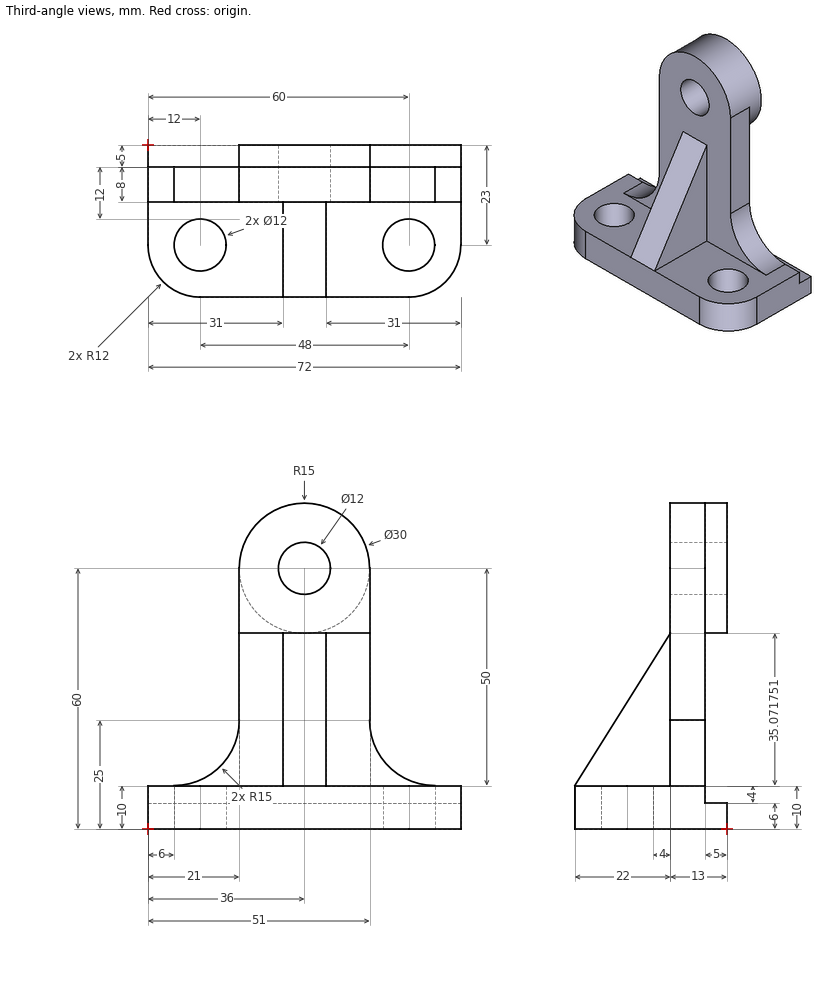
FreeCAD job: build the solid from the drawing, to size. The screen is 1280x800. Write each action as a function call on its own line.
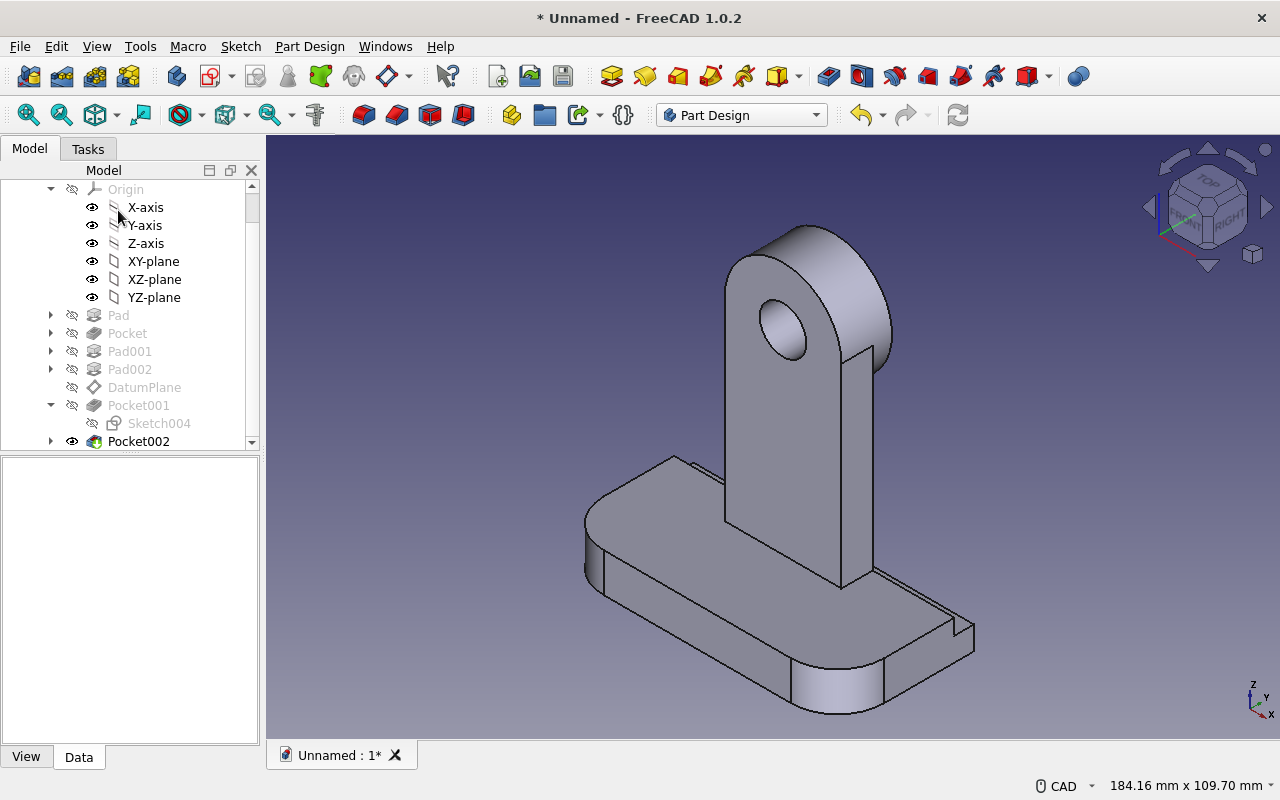
click(783, 449)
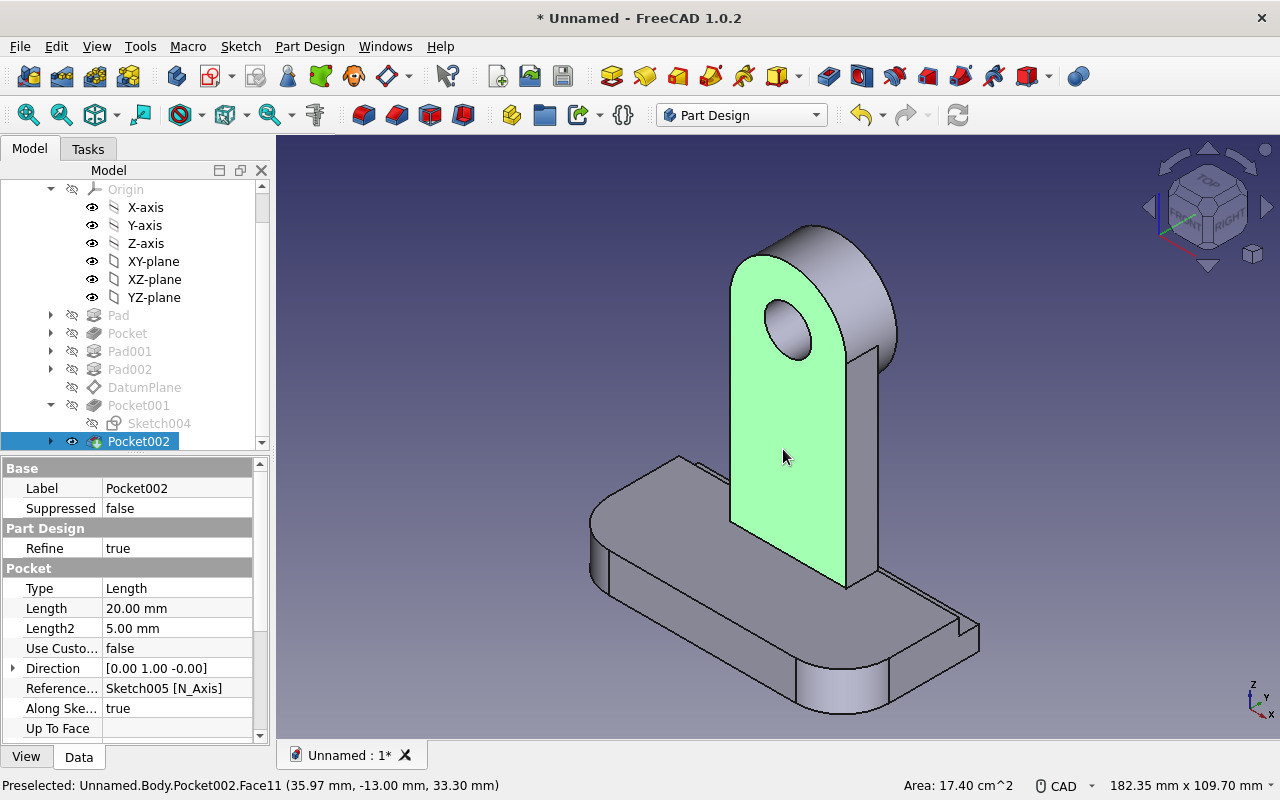
click(210, 76)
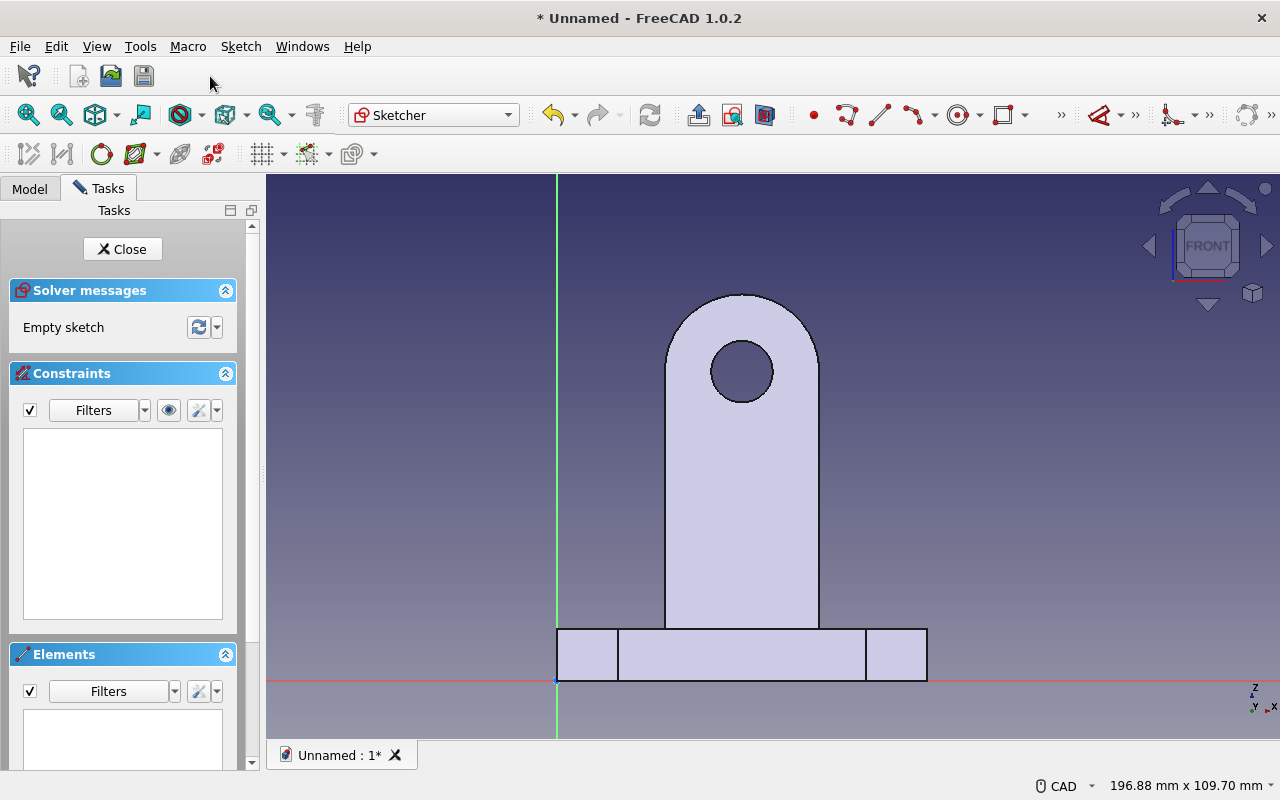
key(q)
key(s)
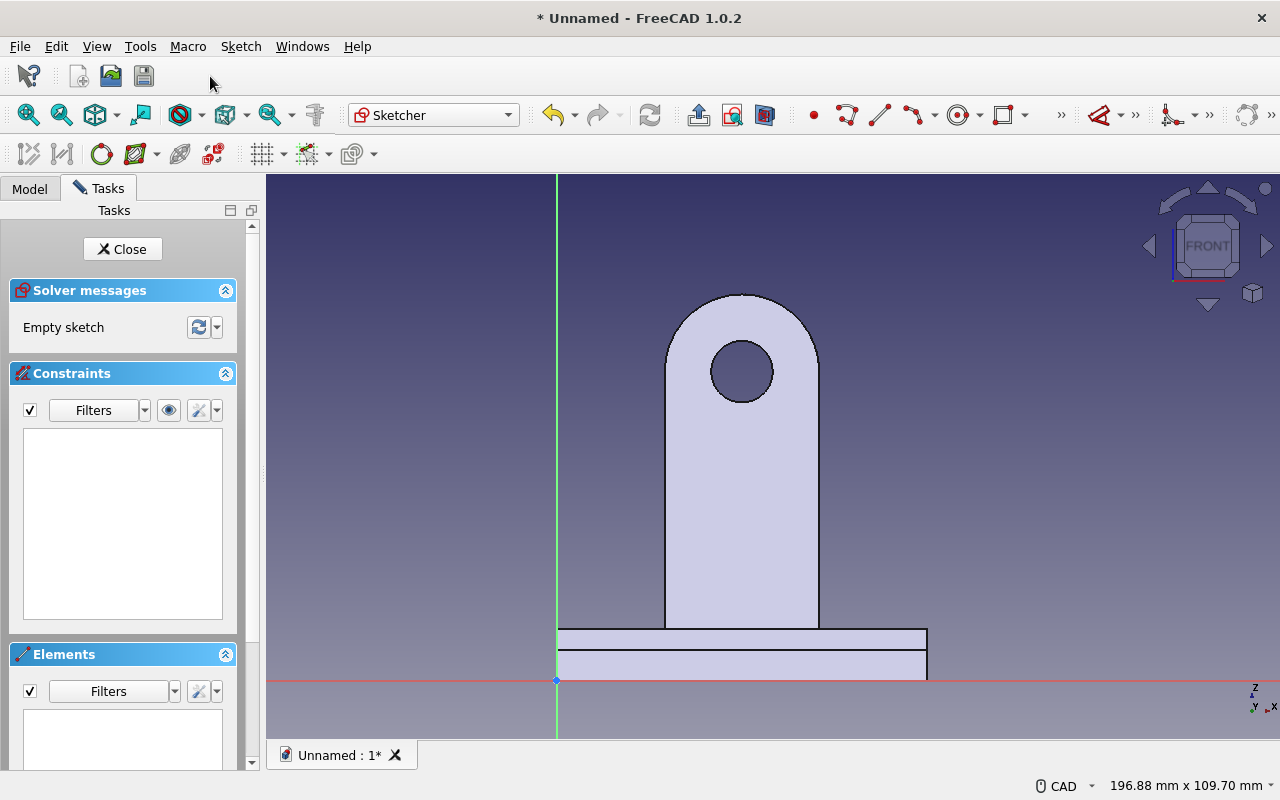
scroll(753, 711, up, 3)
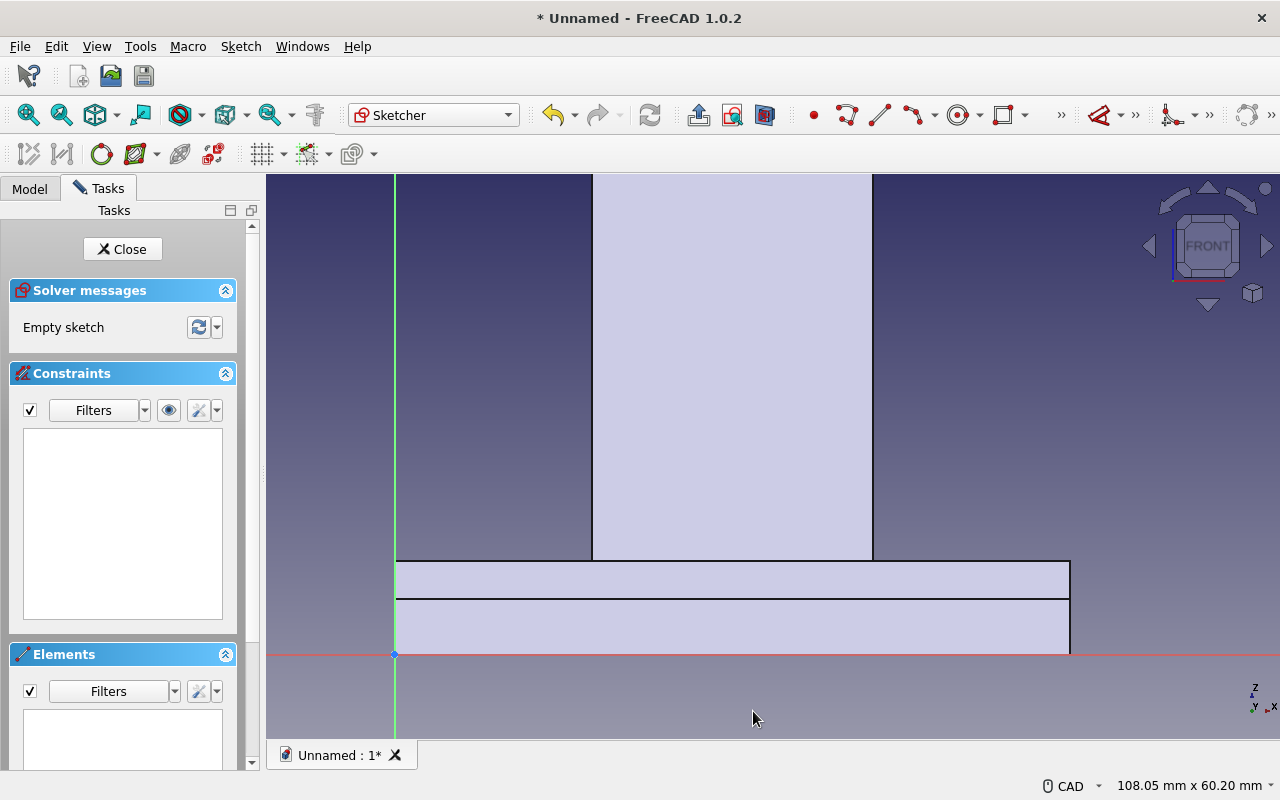
click(847, 116)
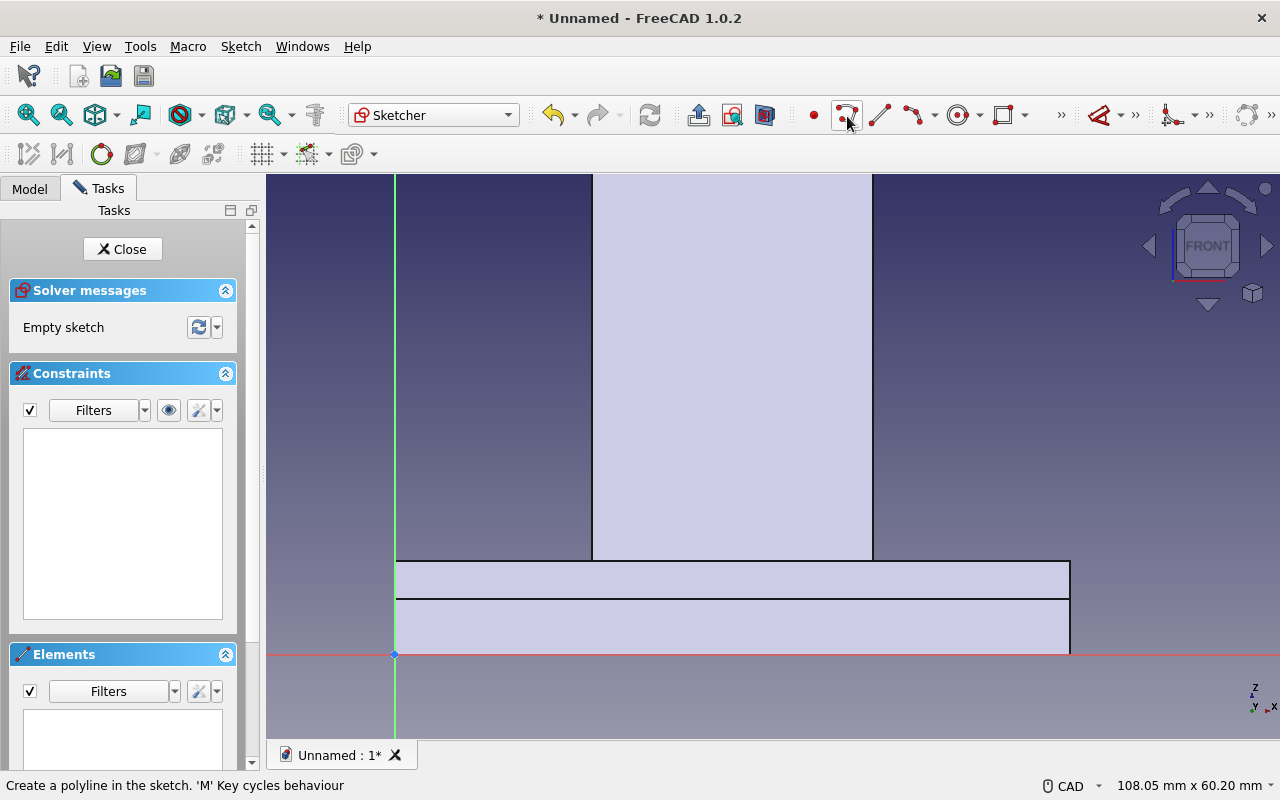
click(451, 561)
click(592, 561)
click(592, 420)
right_click(592, 420)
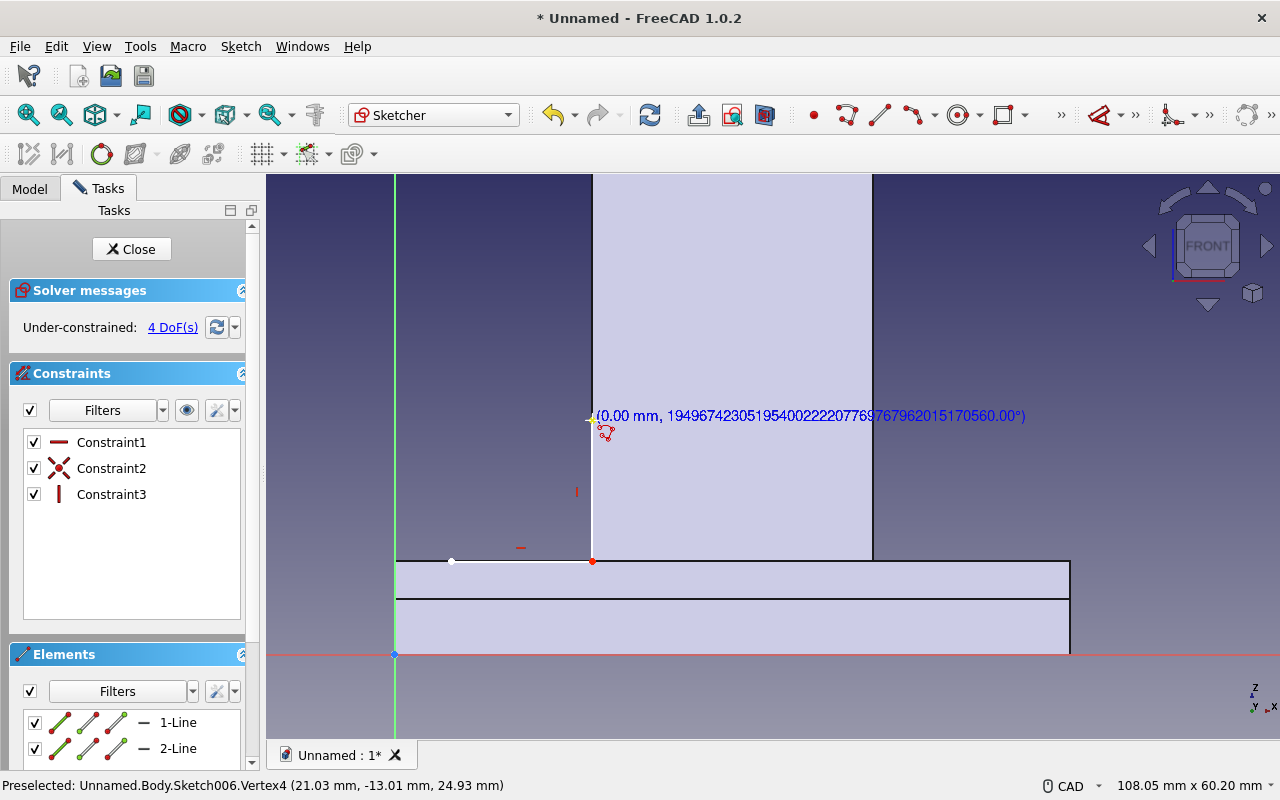
key(g)
key(3)
key(a)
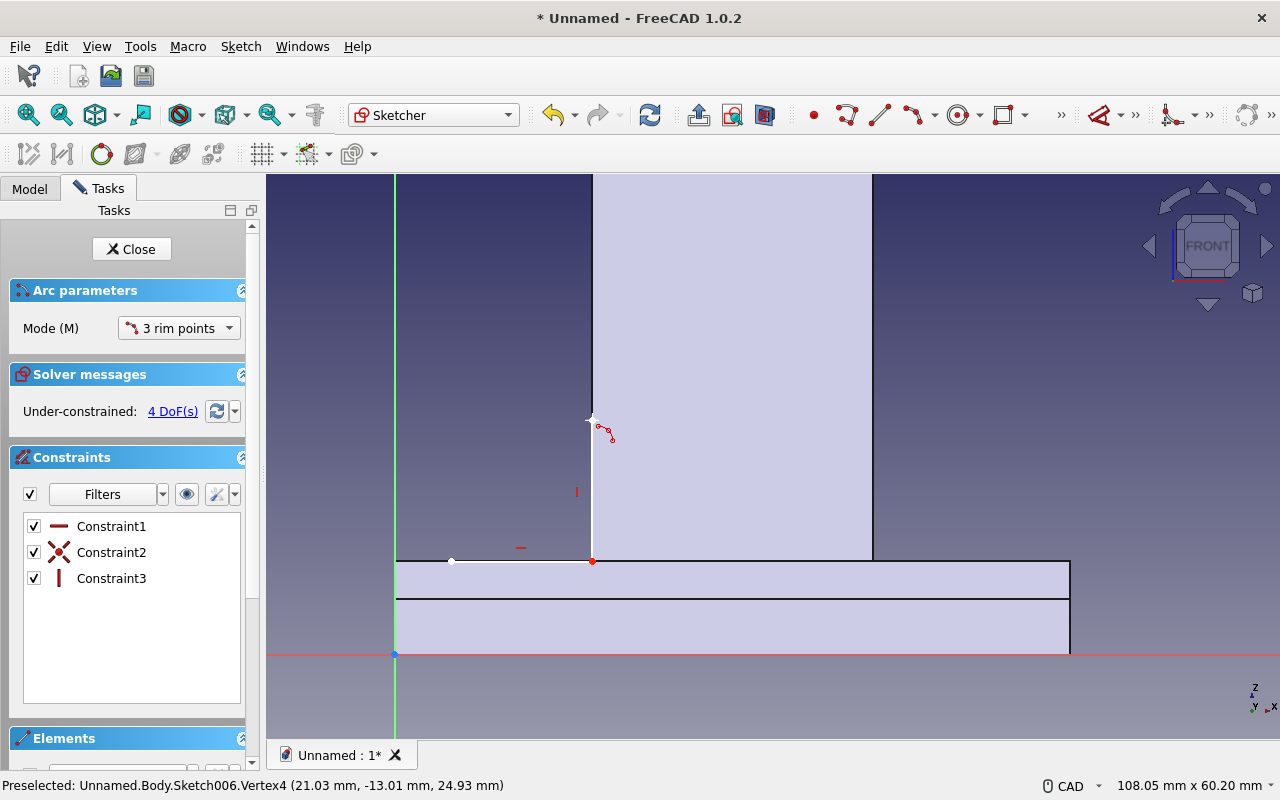
click(592, 421)
click(451, 562)
click(551, 520)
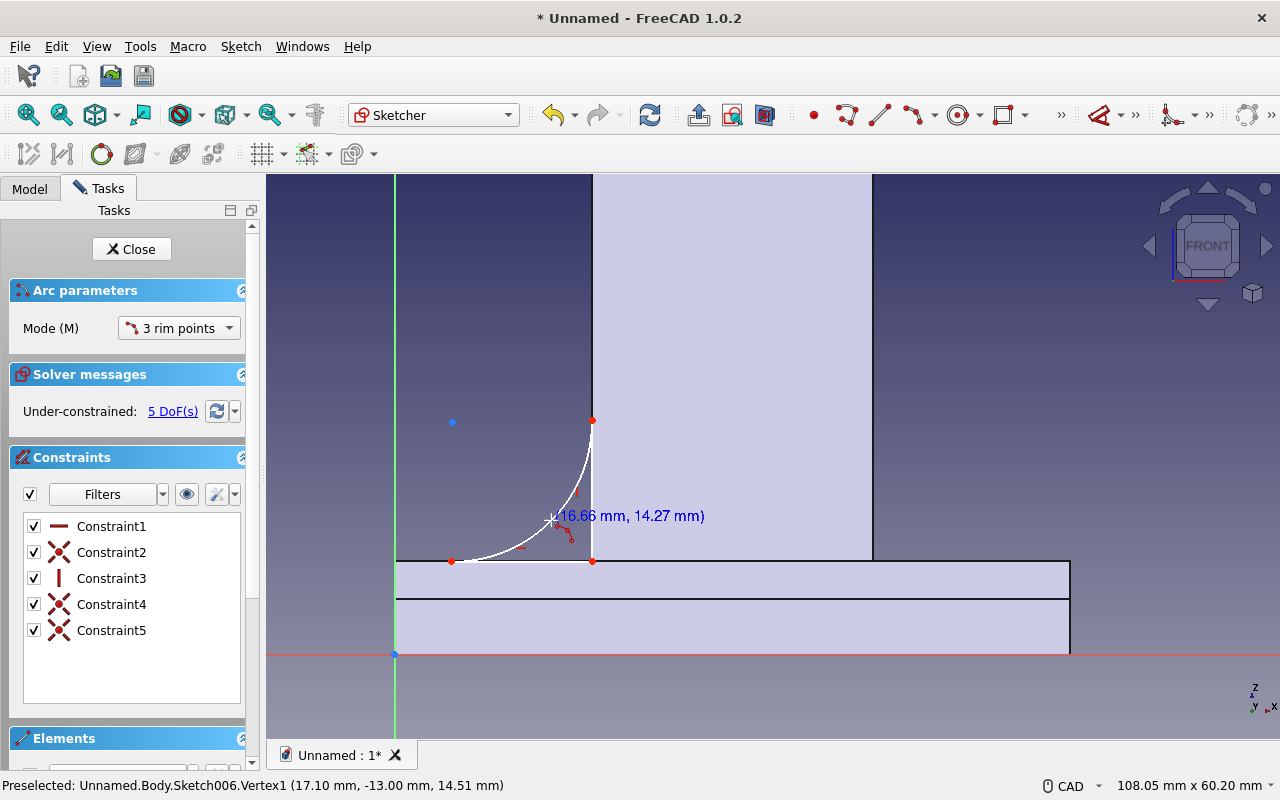
key(g)
key(m)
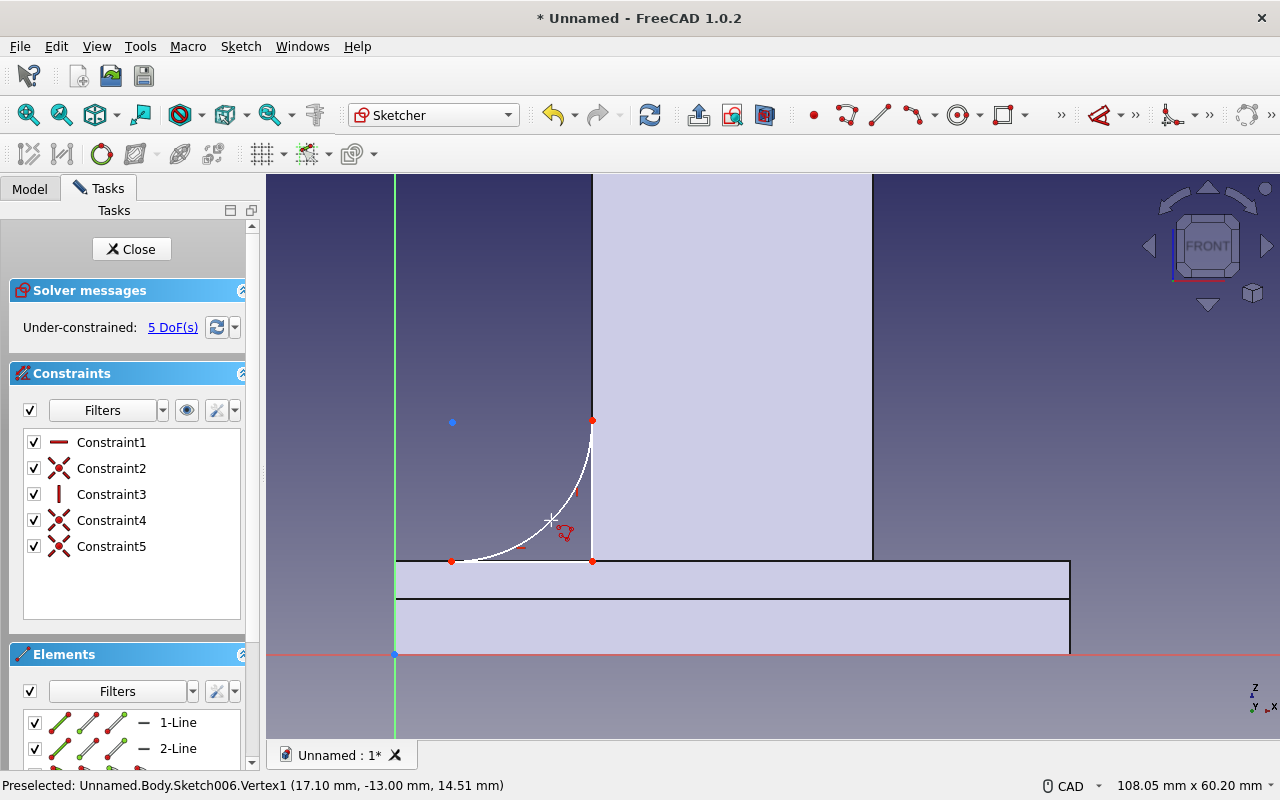
click(873, 420)
click(873, 561)
click(1014, 561)
right_click(1014, 561)